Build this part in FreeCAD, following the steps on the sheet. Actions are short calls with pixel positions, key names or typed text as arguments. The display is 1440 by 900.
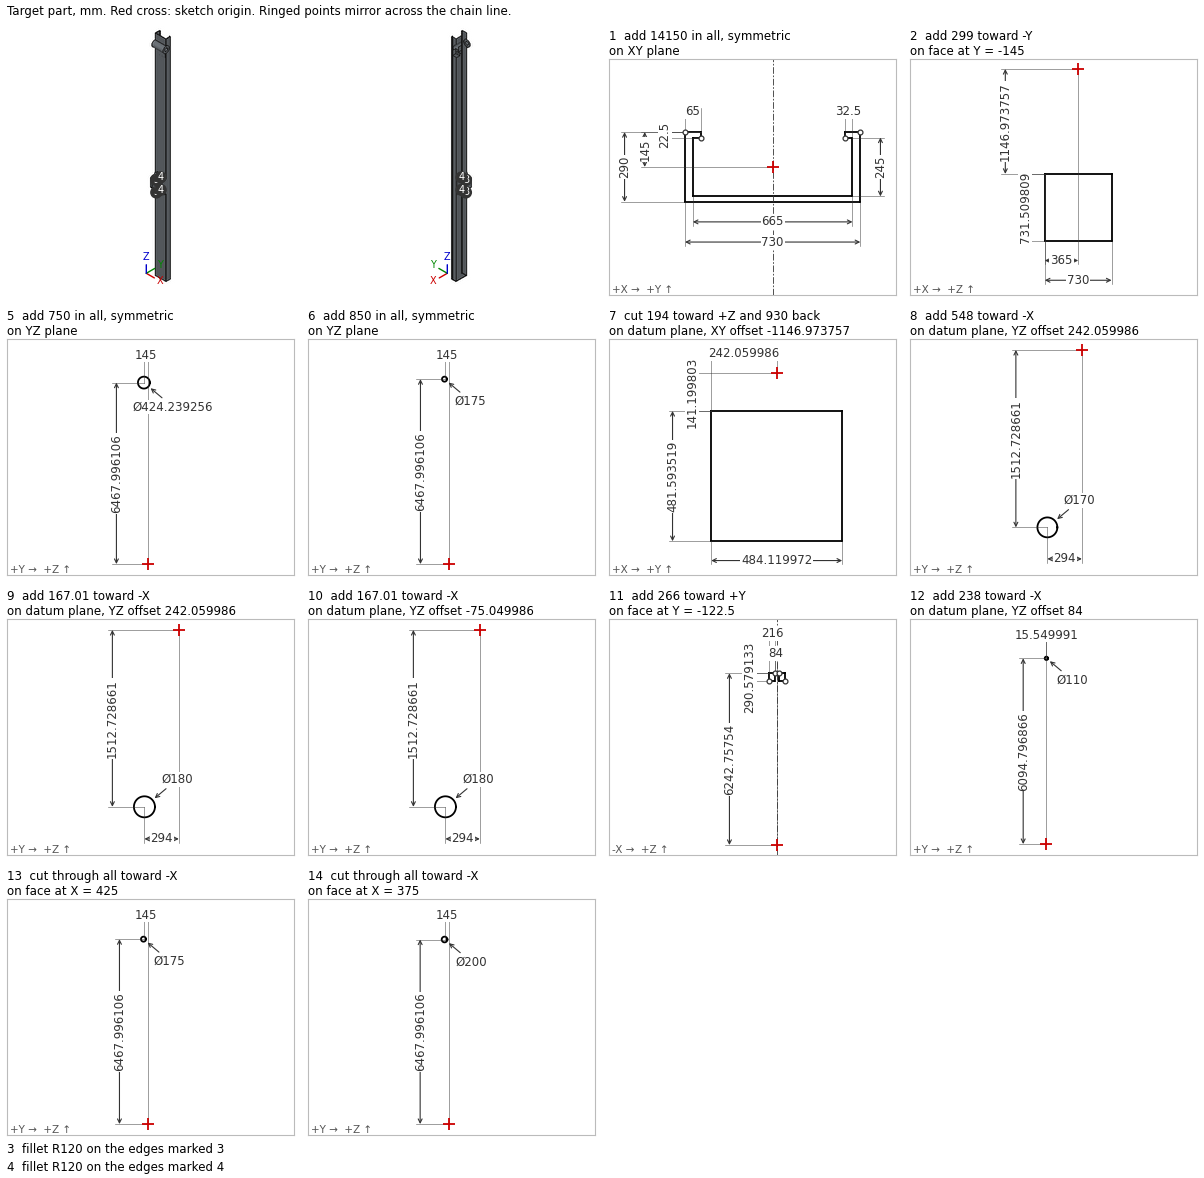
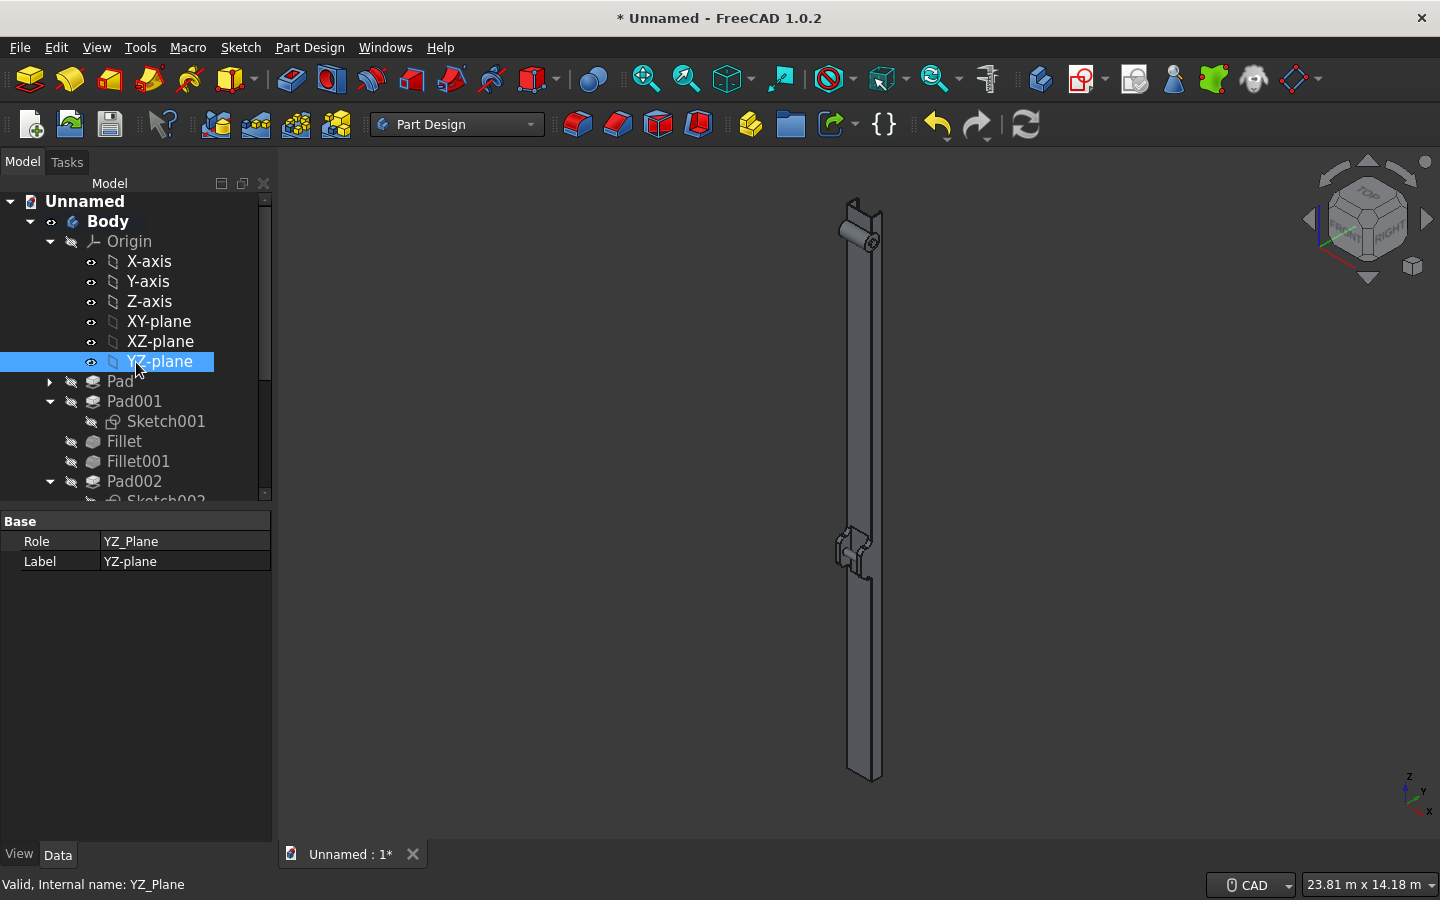
click(1294, 80)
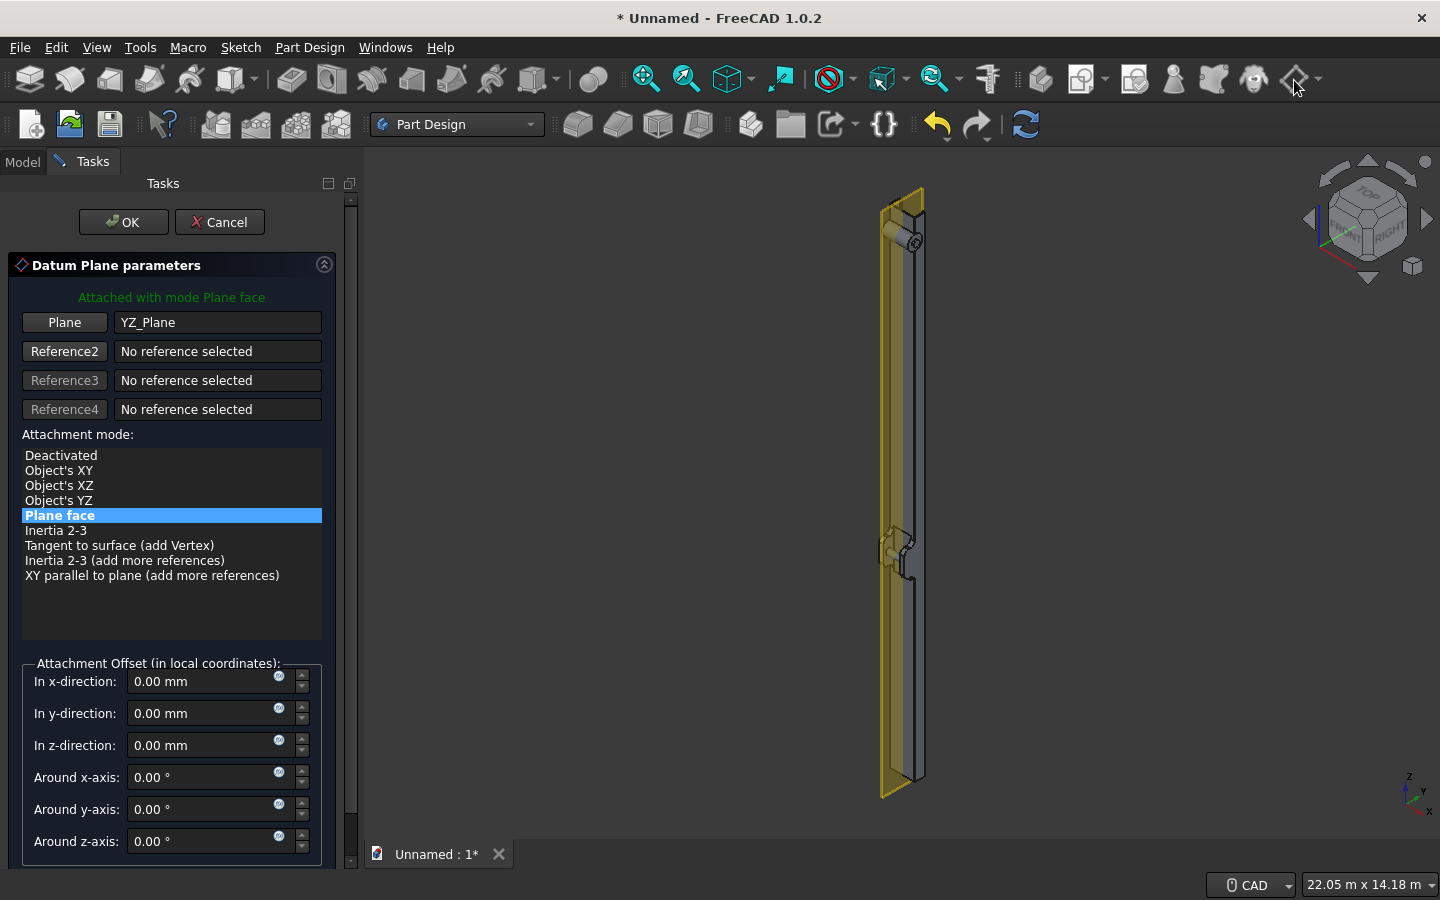
triple_click(210, 745)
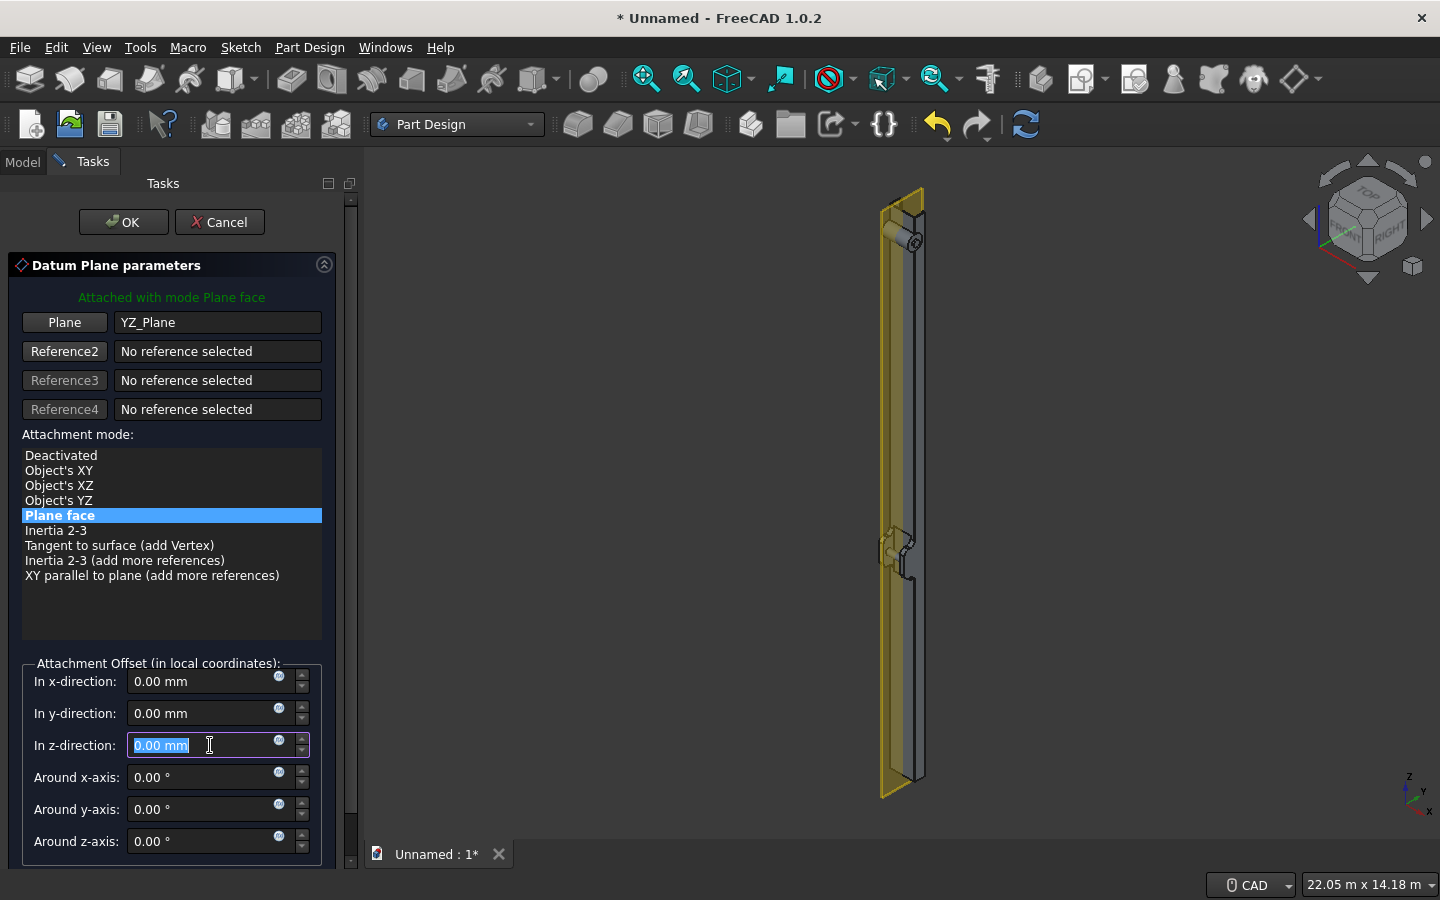
text(242.059986)
key(Tab)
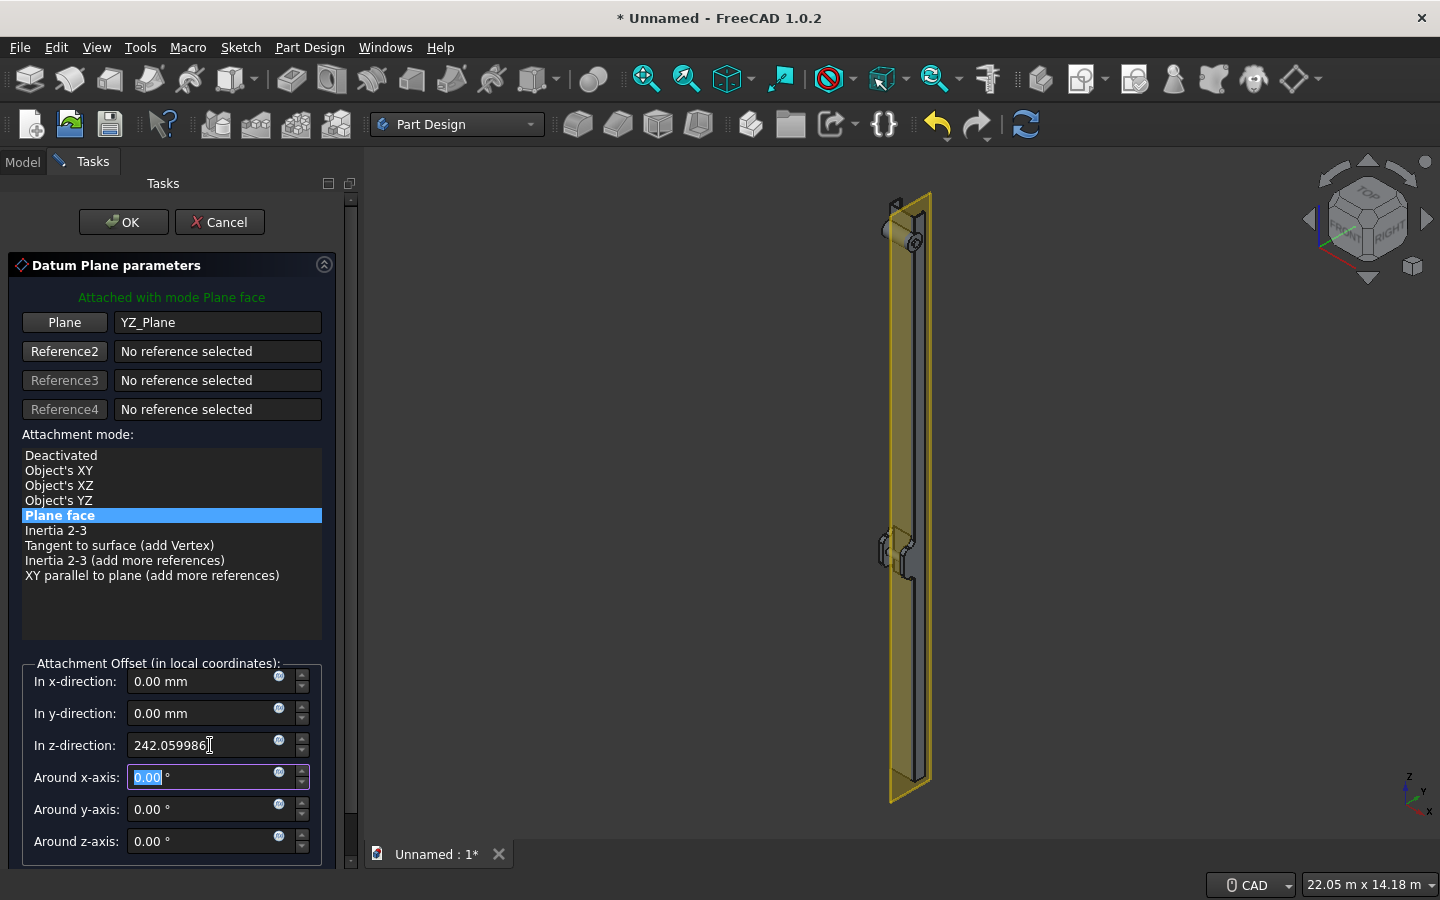
click(124, 222)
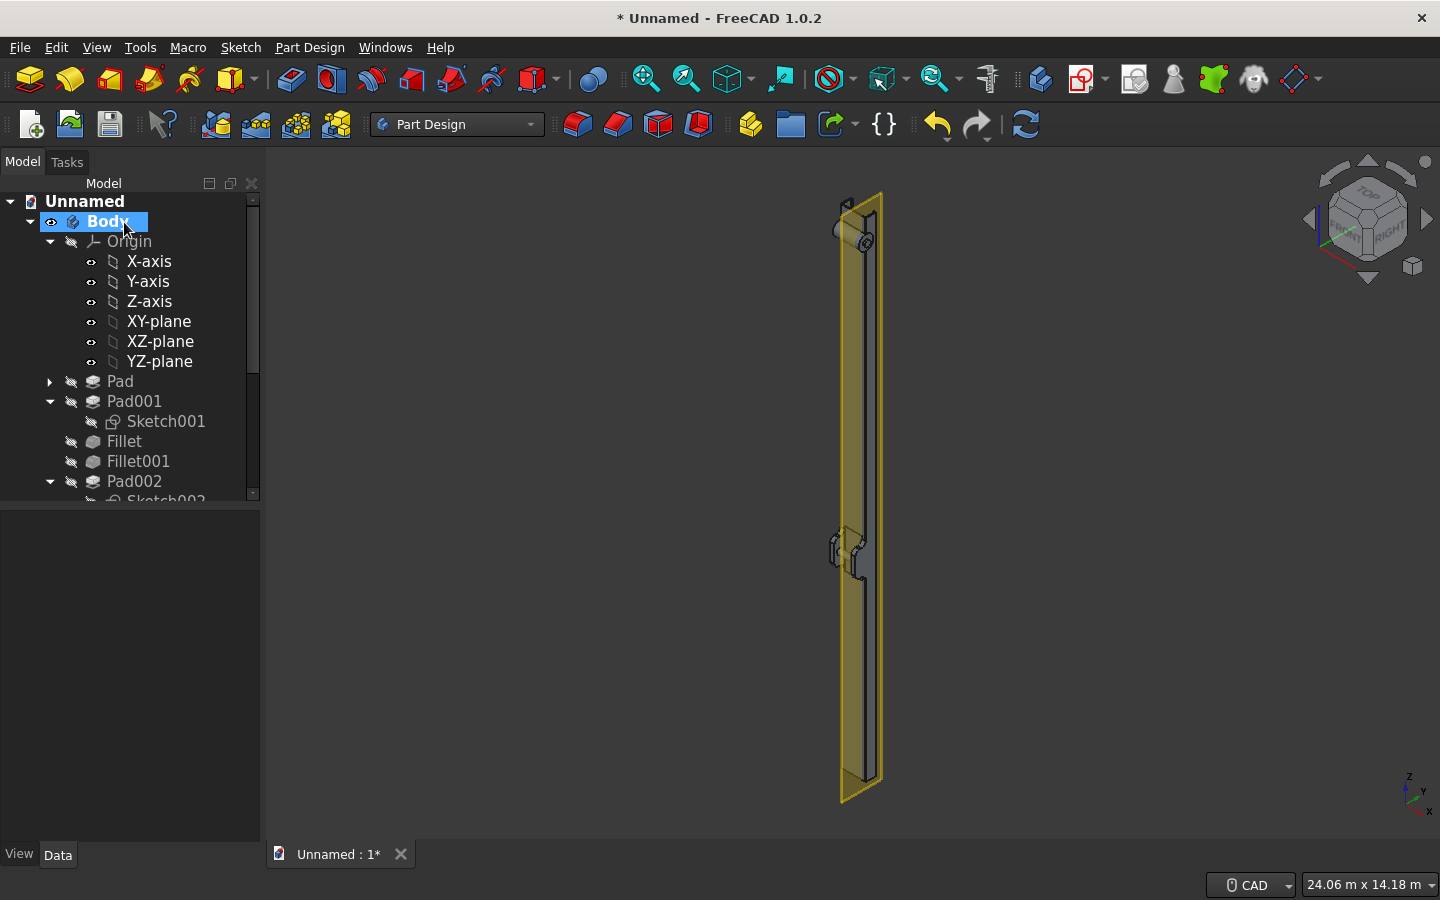
scroll(100, 337, down, 3)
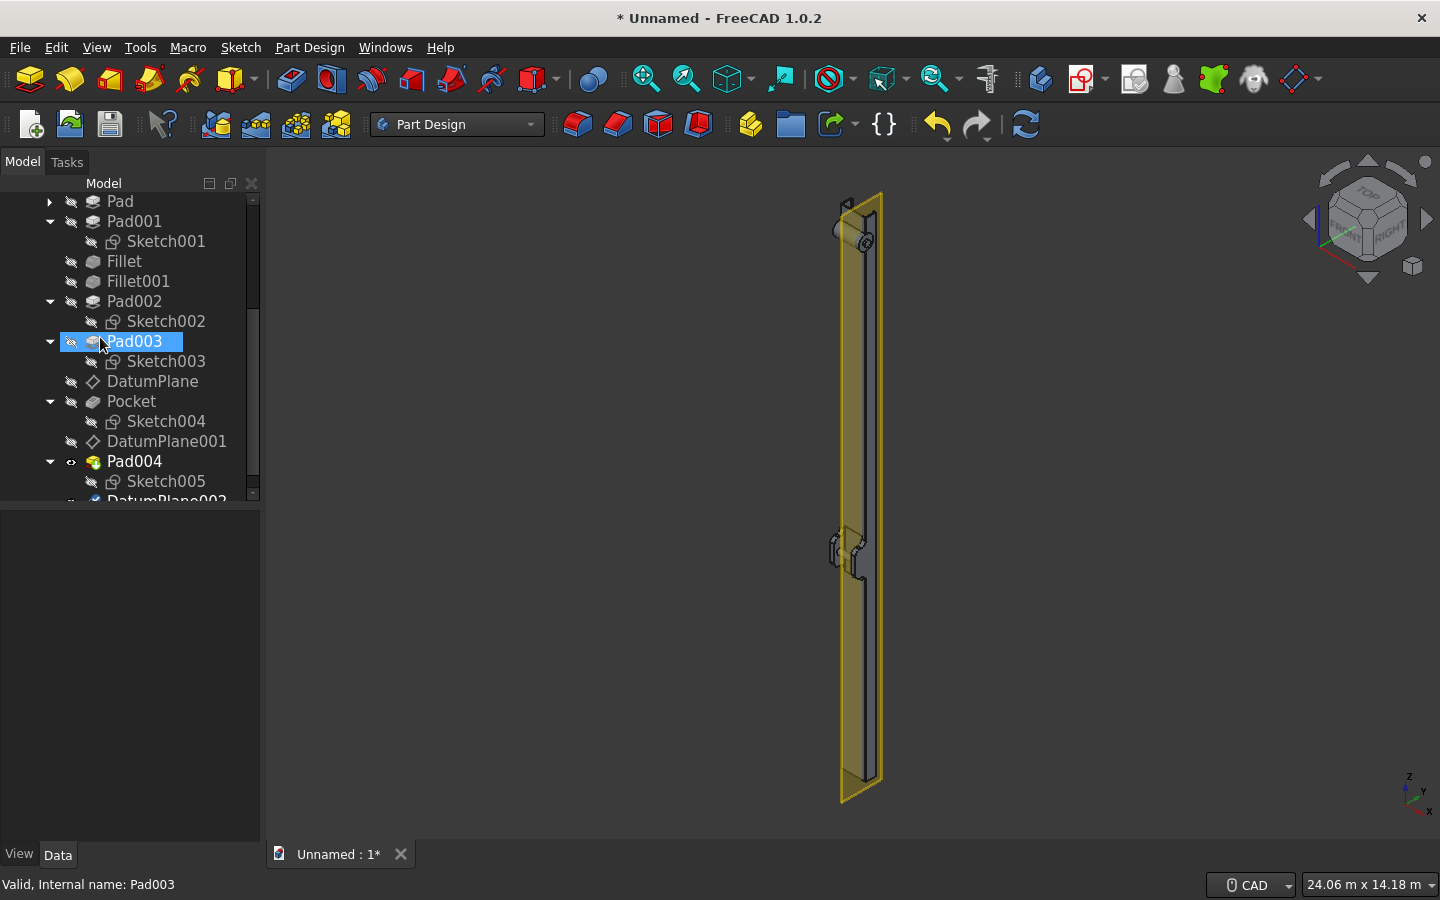
scroll(140, 337, up, 15)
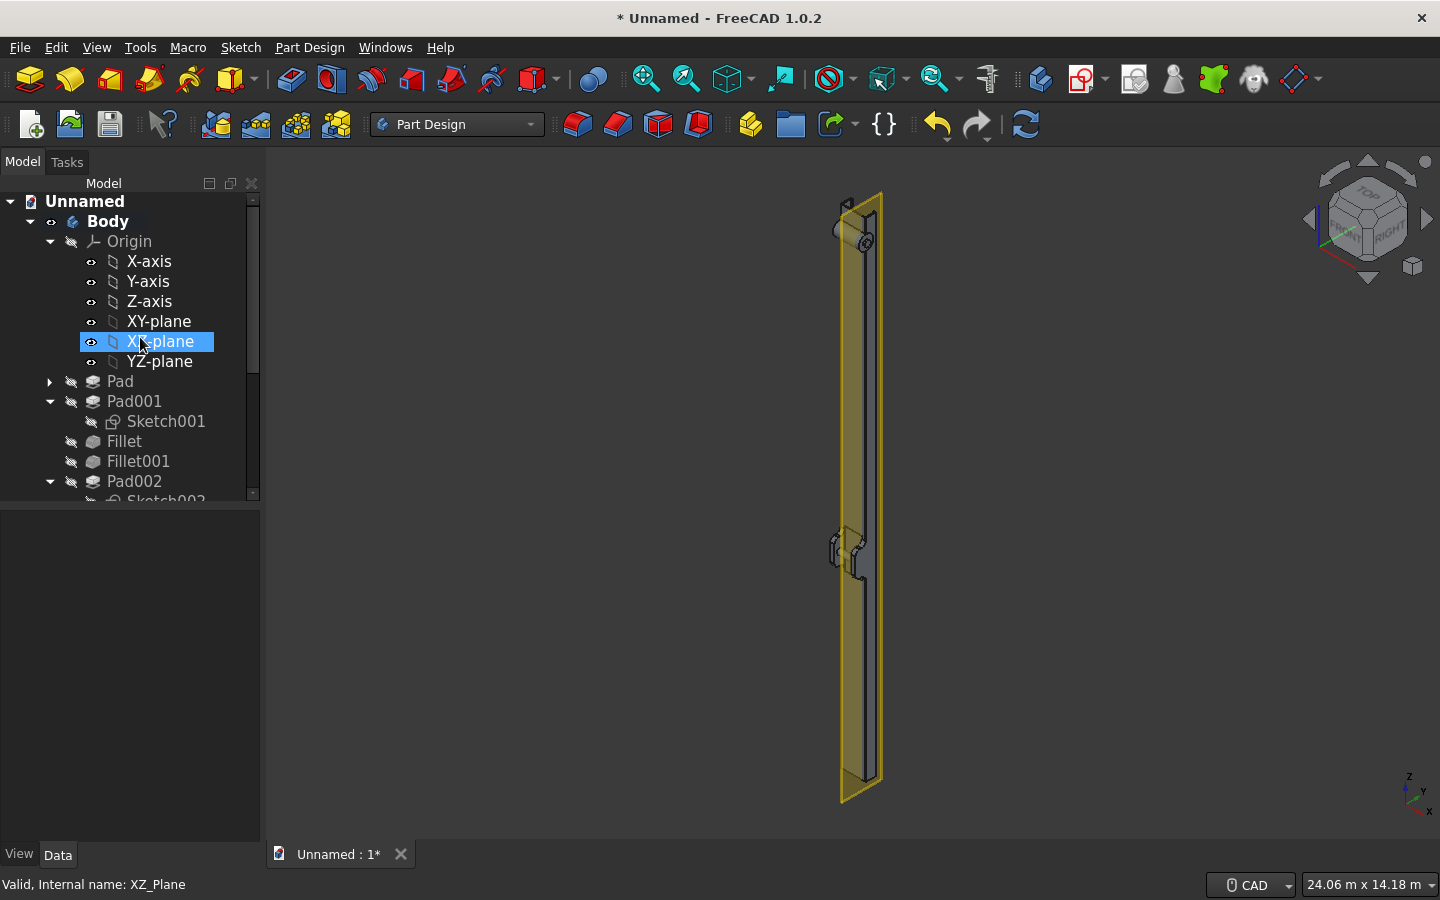
scroll(100, 337, down, 6)